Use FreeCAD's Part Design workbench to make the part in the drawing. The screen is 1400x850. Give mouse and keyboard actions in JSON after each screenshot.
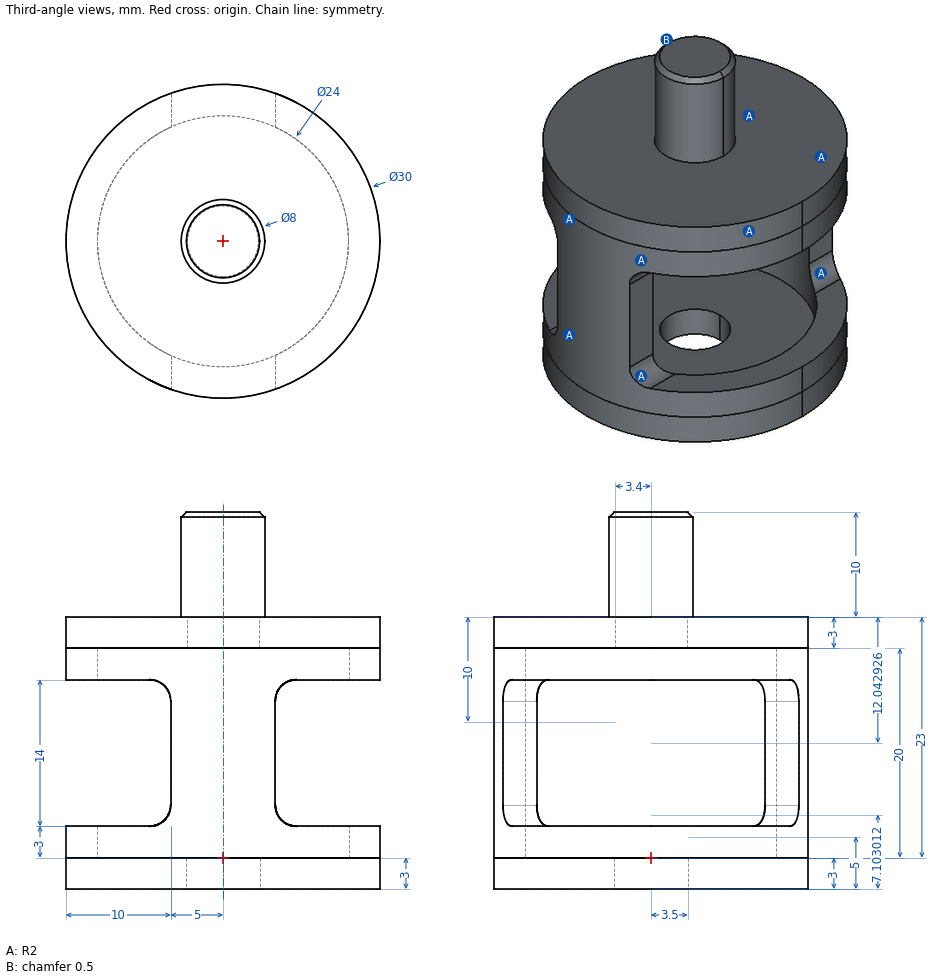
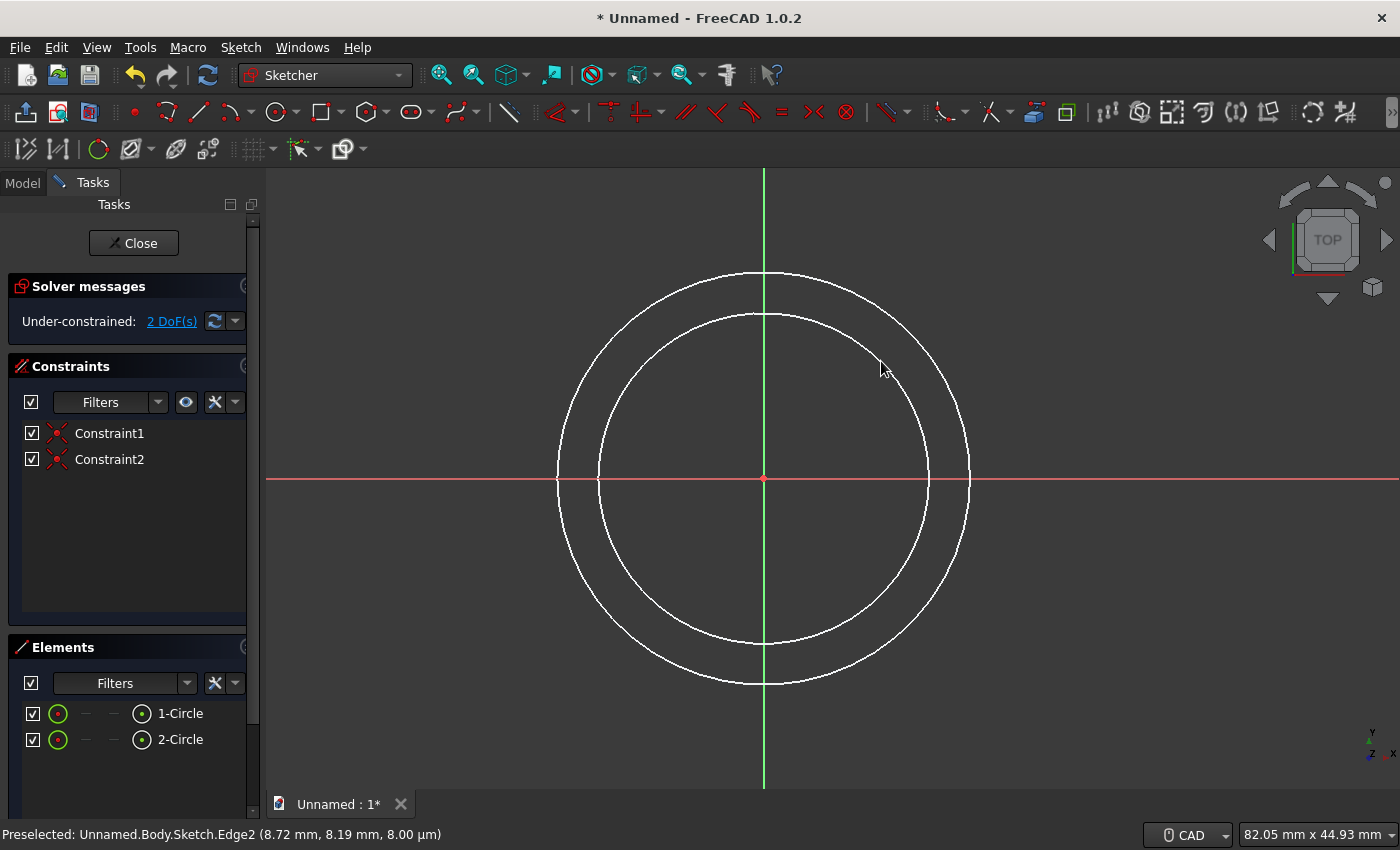
{"action": "left_click", "coordinate": [909, 332]}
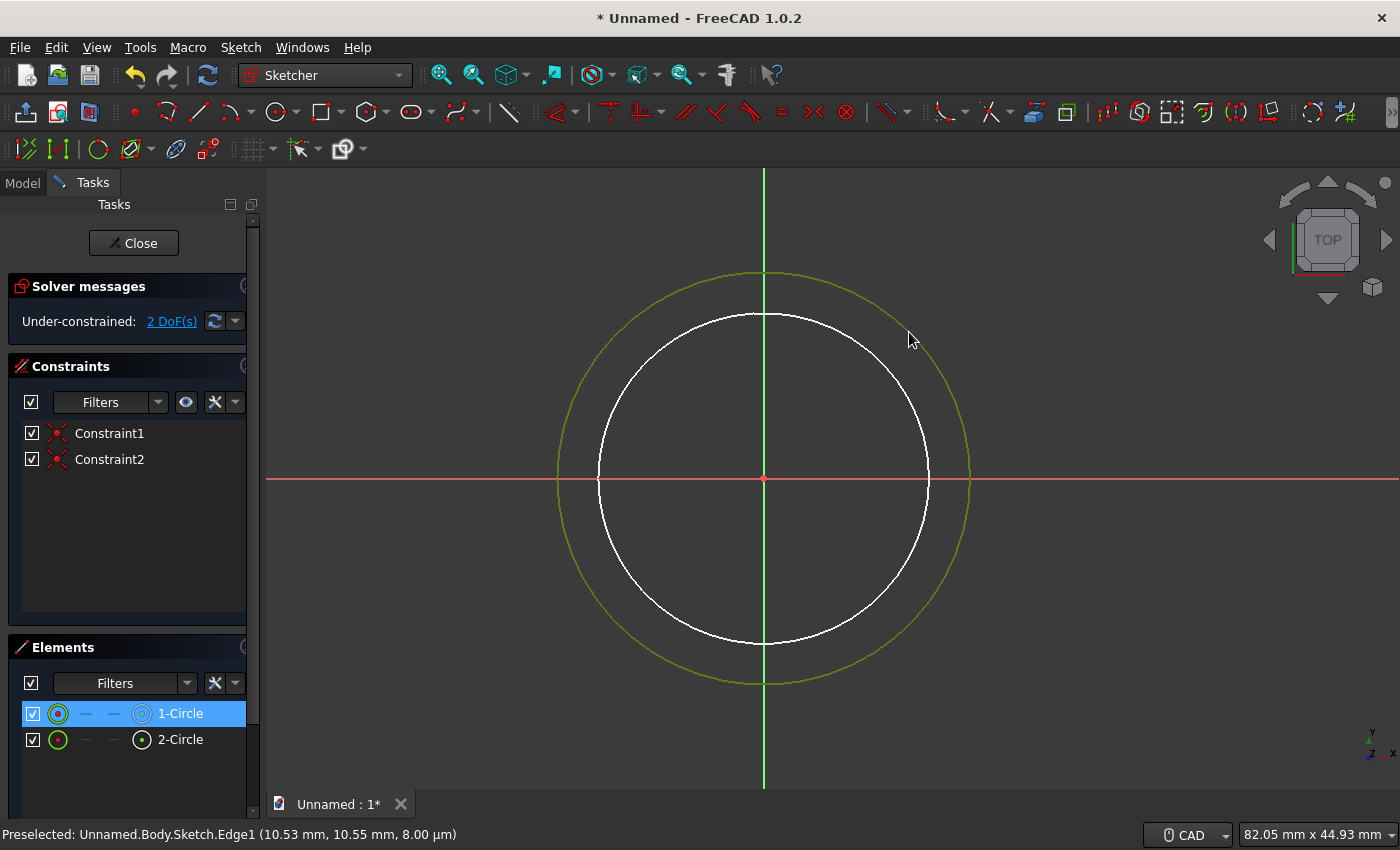
{"action": "left_click", "coordinate": [578, 112]}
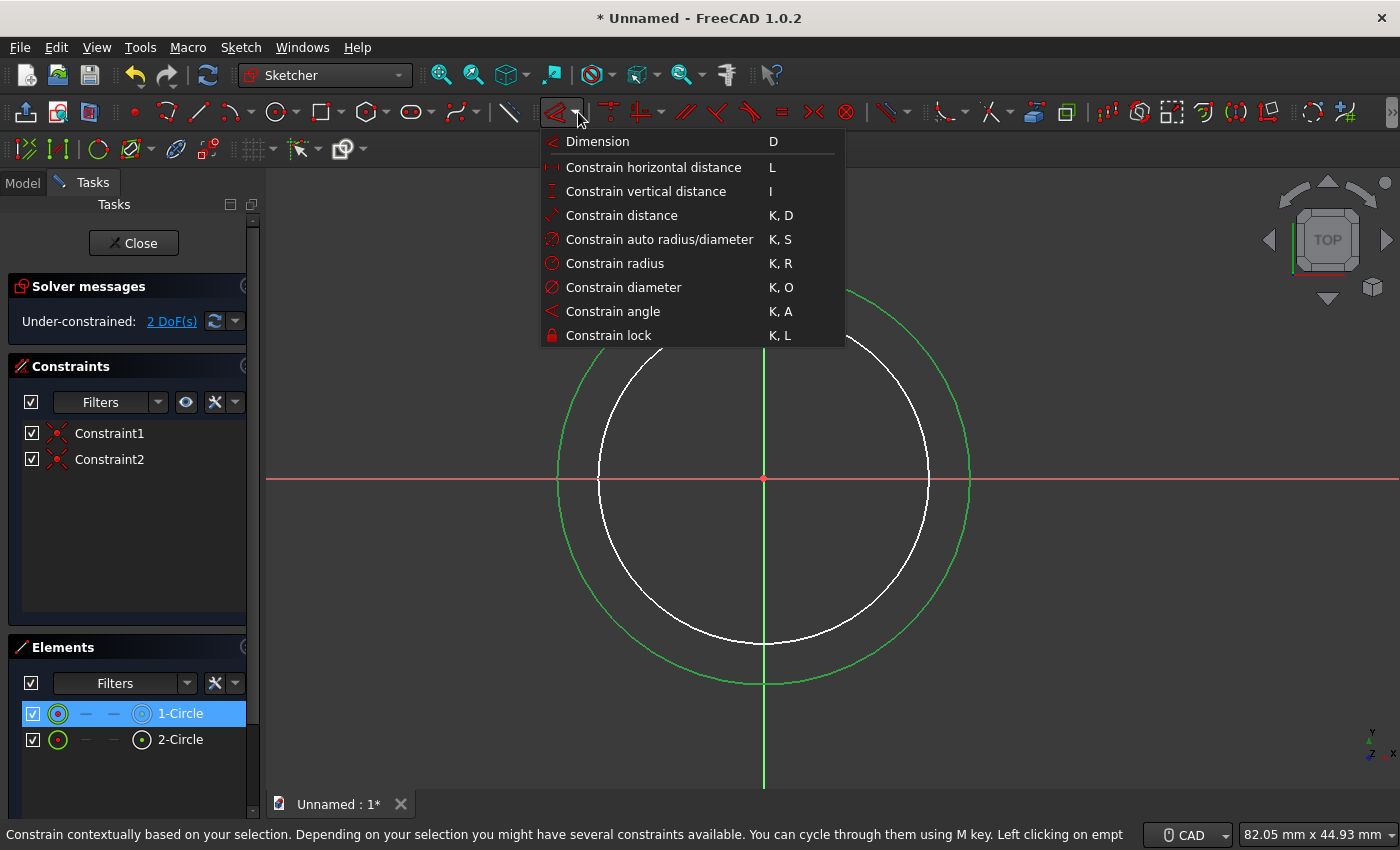
{"action": "left_click", "coordinate": [693, 287]}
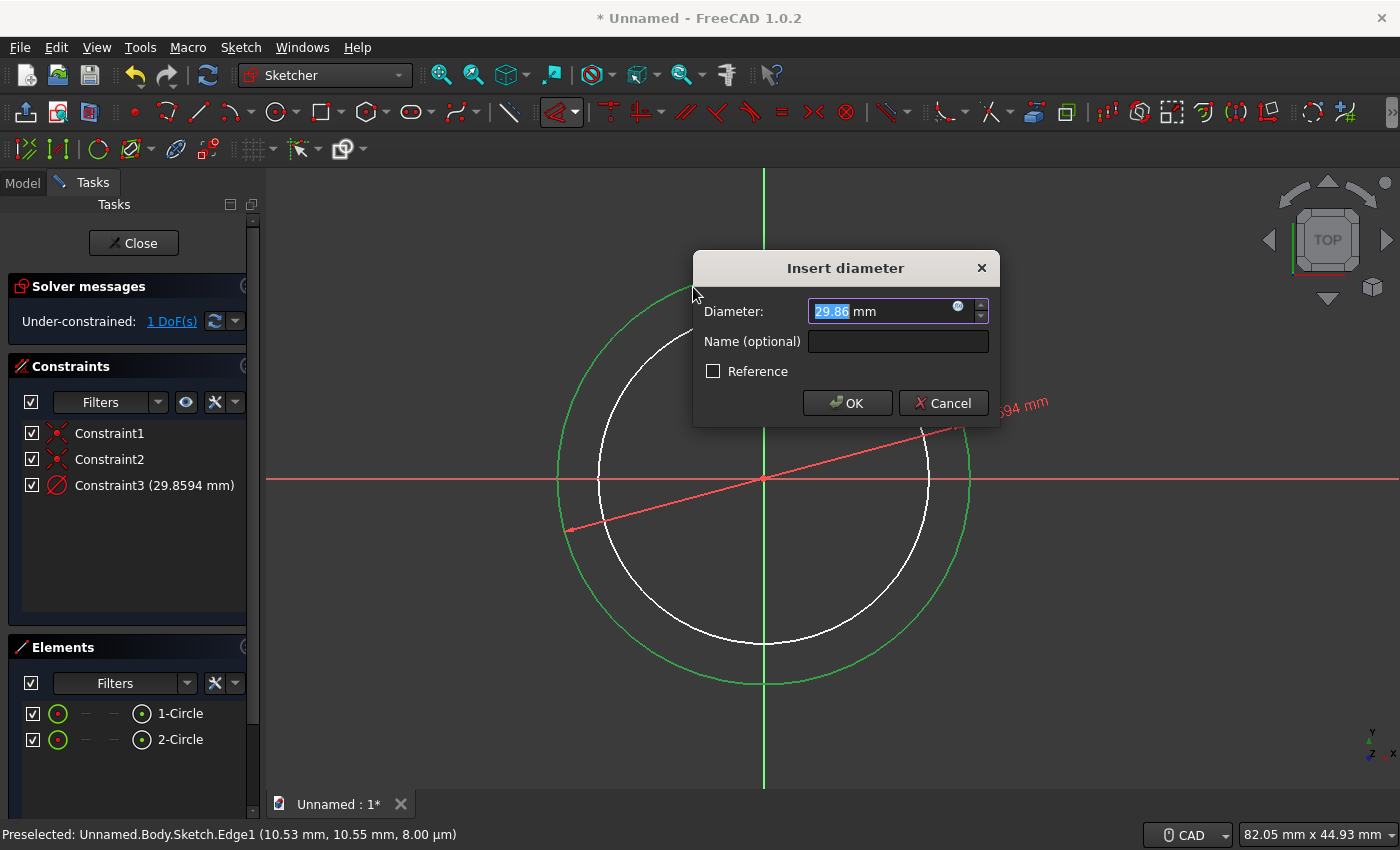
{"action": "type", "text": "30"}
{"action": "key", "text": "Return"}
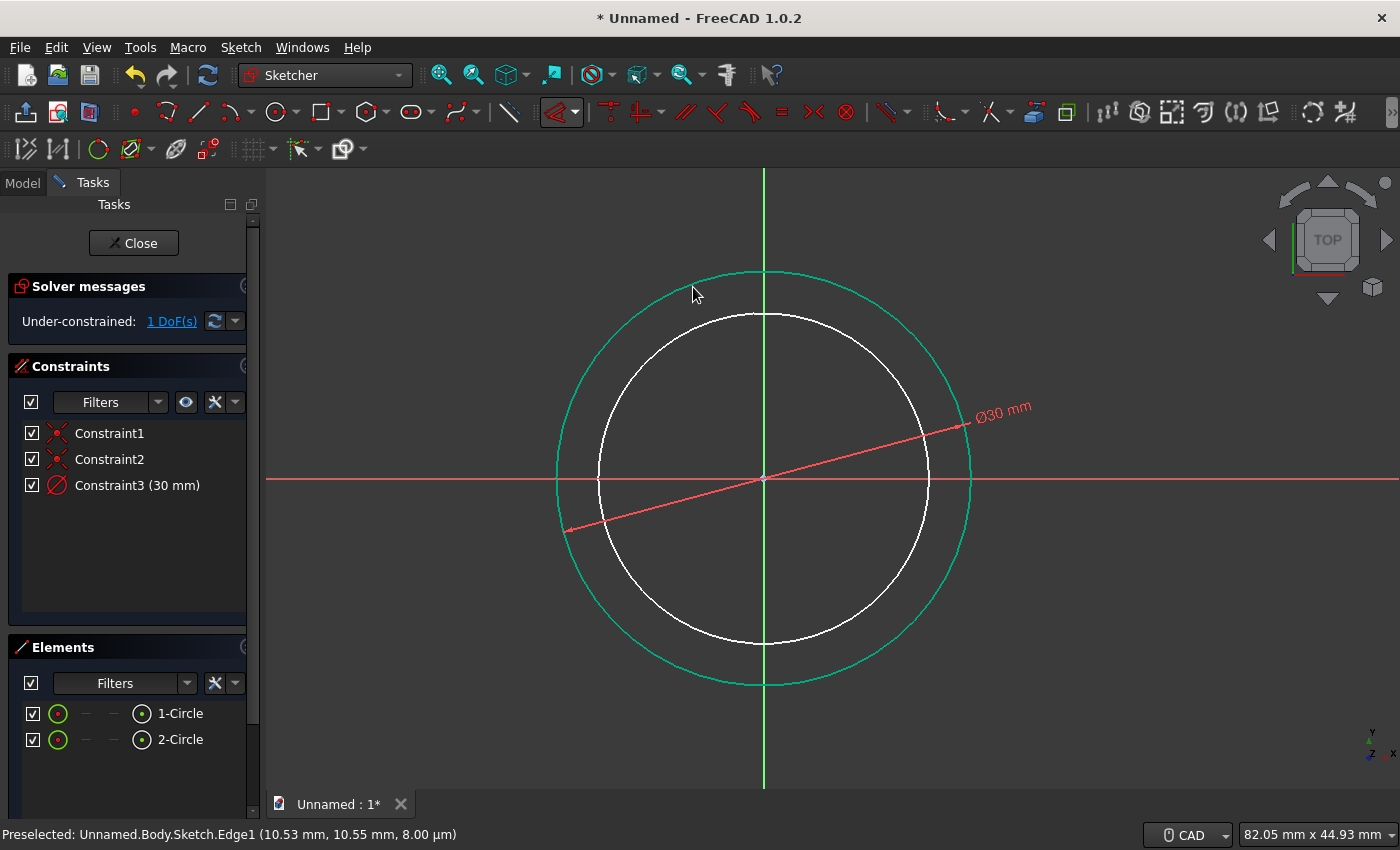
{"action": "left_click", "coordinate": [880, 361]}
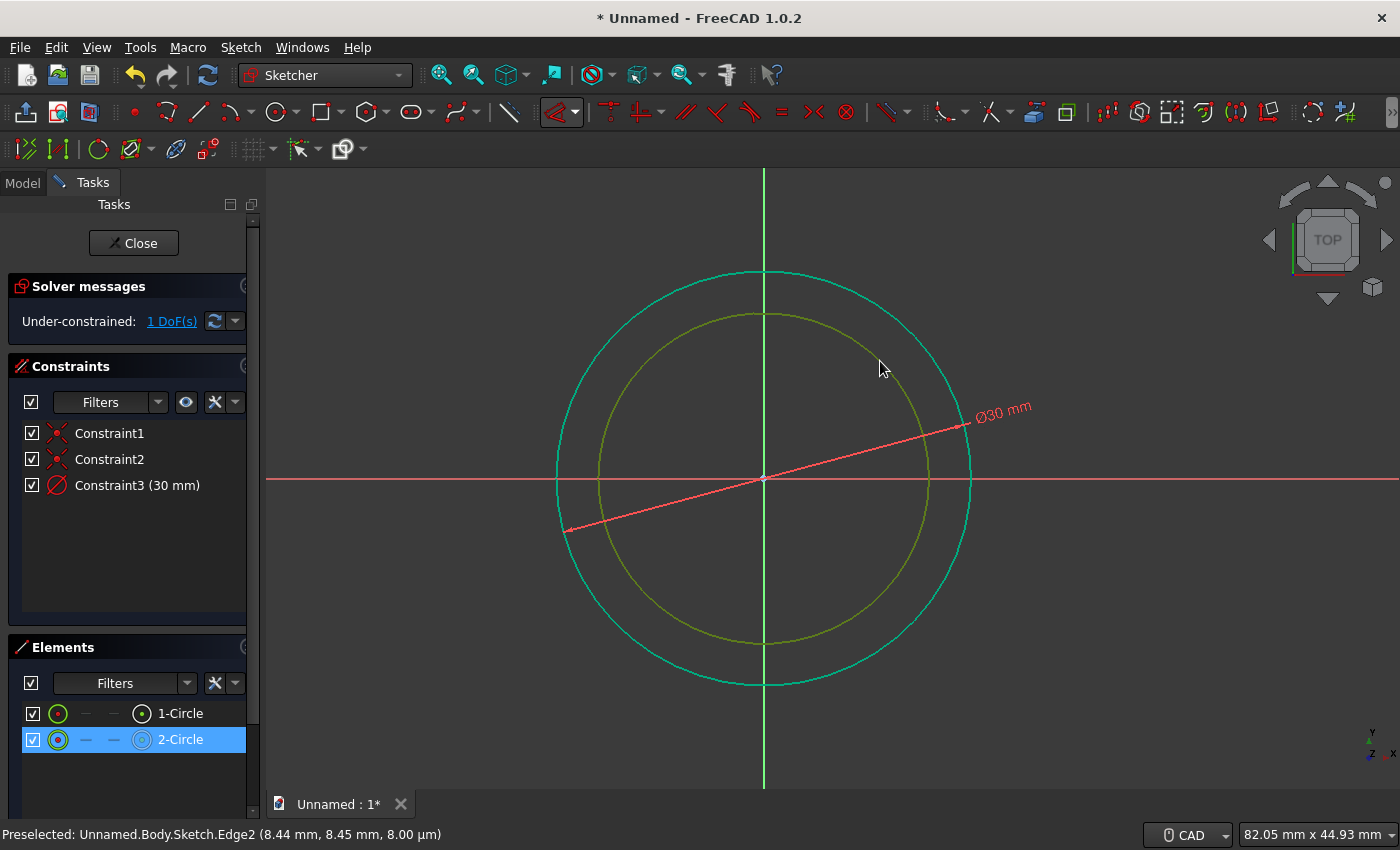
{"action": "left_click", "coordinate": [578, 112]}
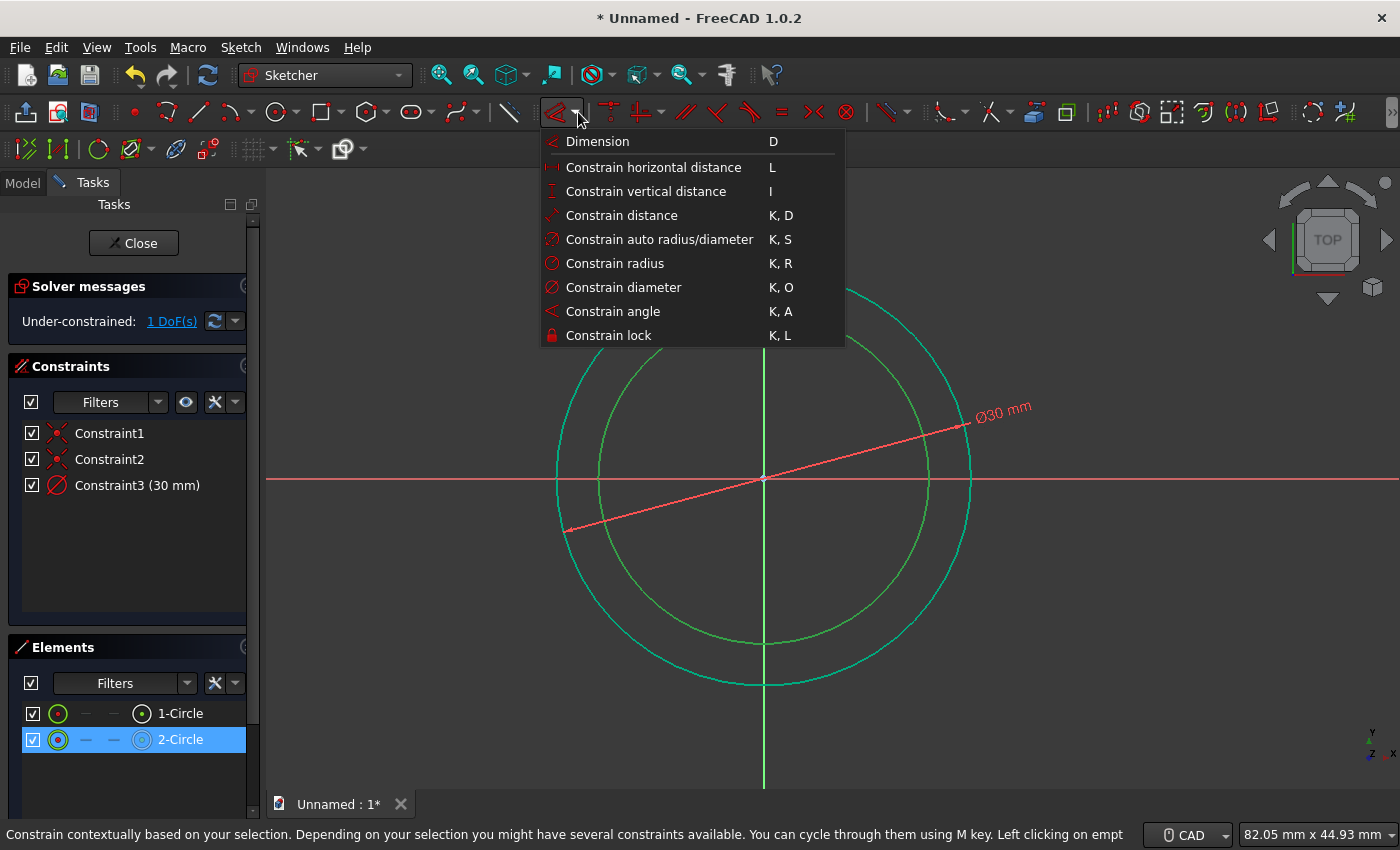
{"action": "left_click", "coordinate": [693, 287]}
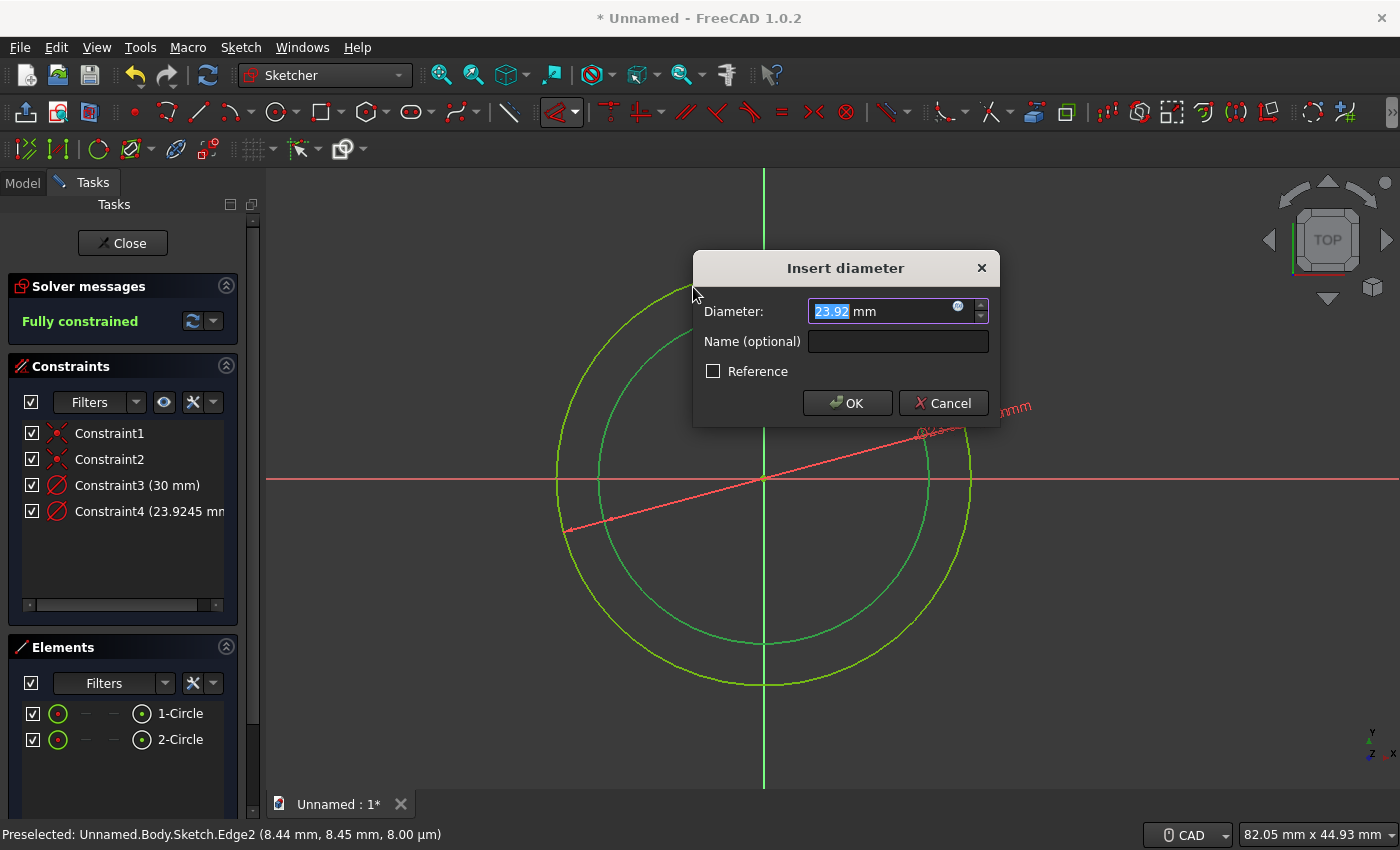
{"action": "type", "text": "24"}
{"action": "key", "text": "Return"}